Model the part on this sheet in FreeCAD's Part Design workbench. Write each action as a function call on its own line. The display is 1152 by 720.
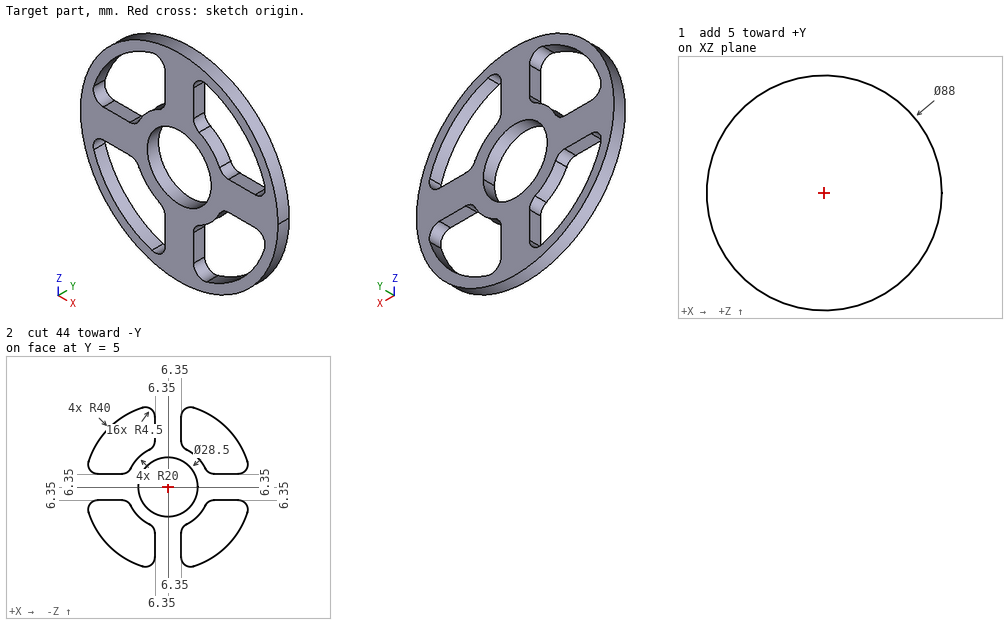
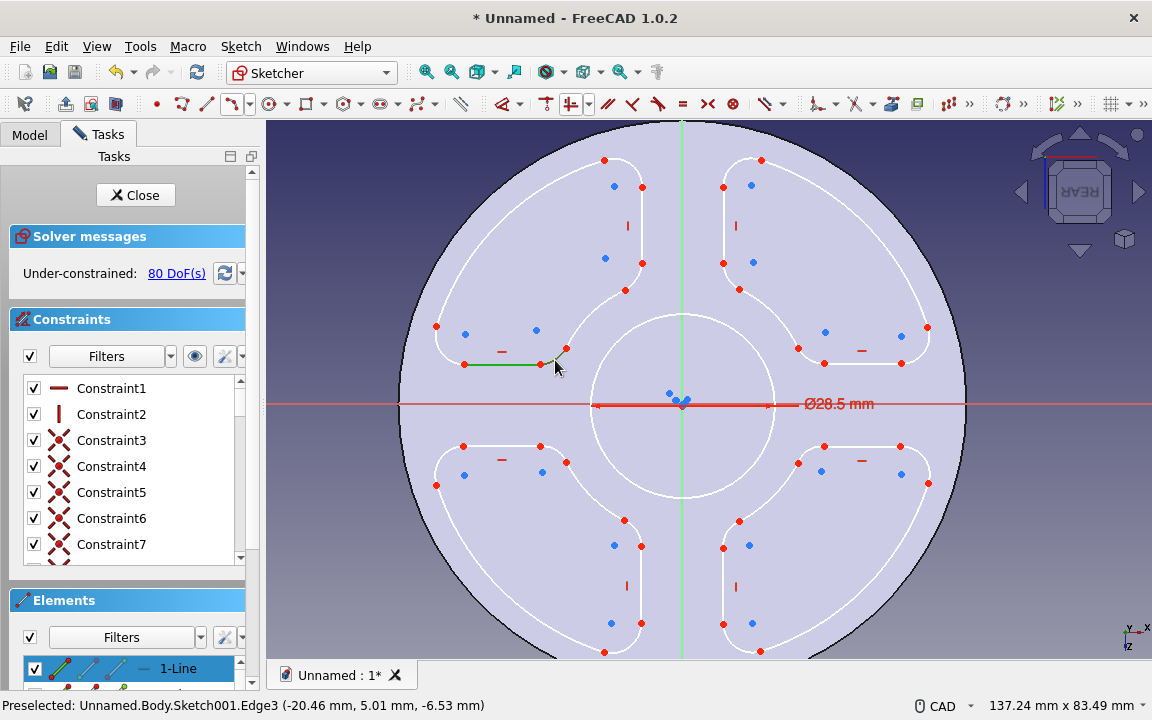
key(t)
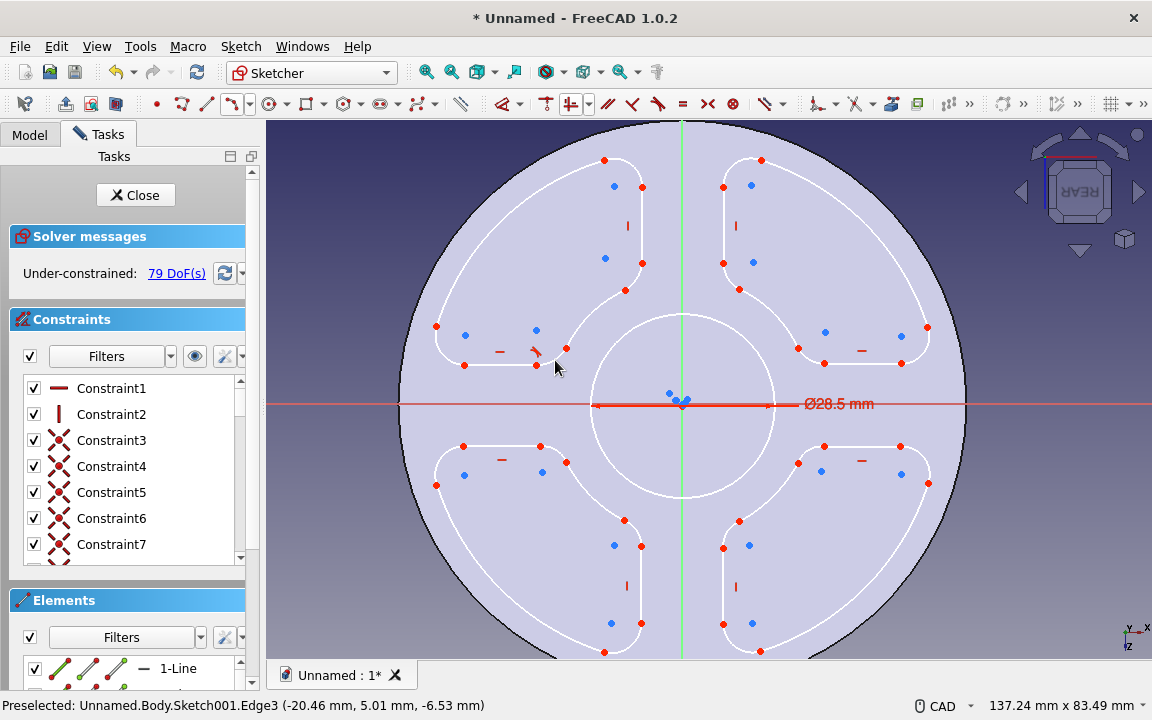
click(486, 365)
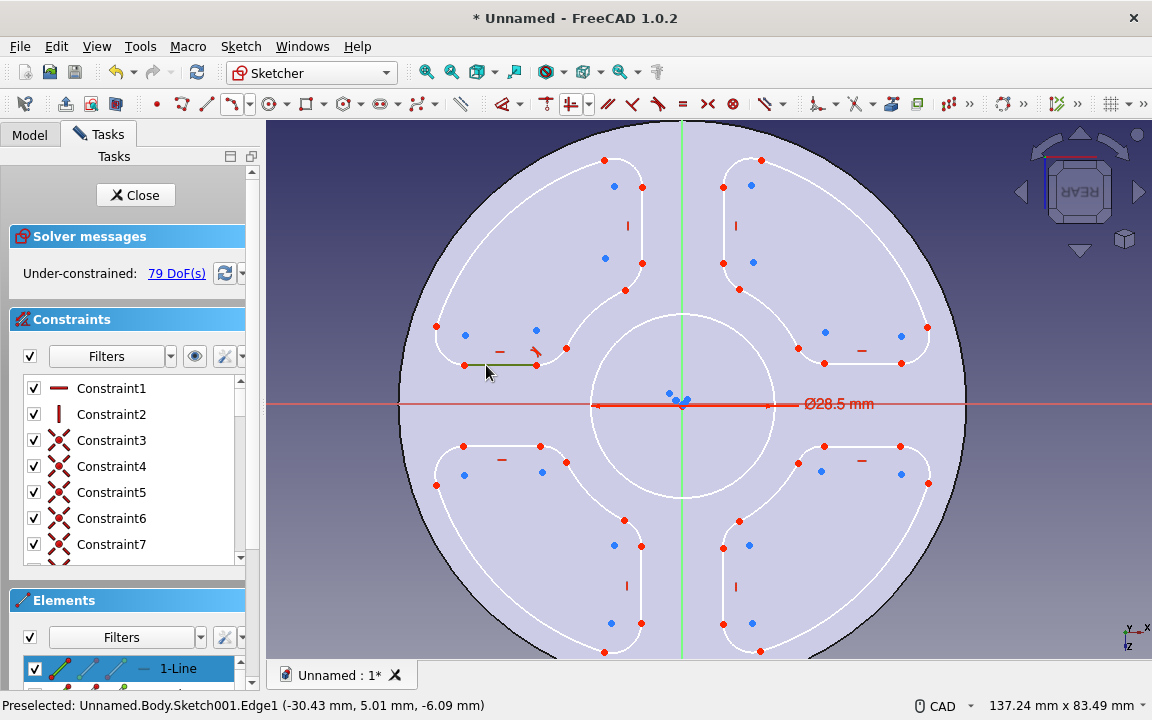
click(437, 343)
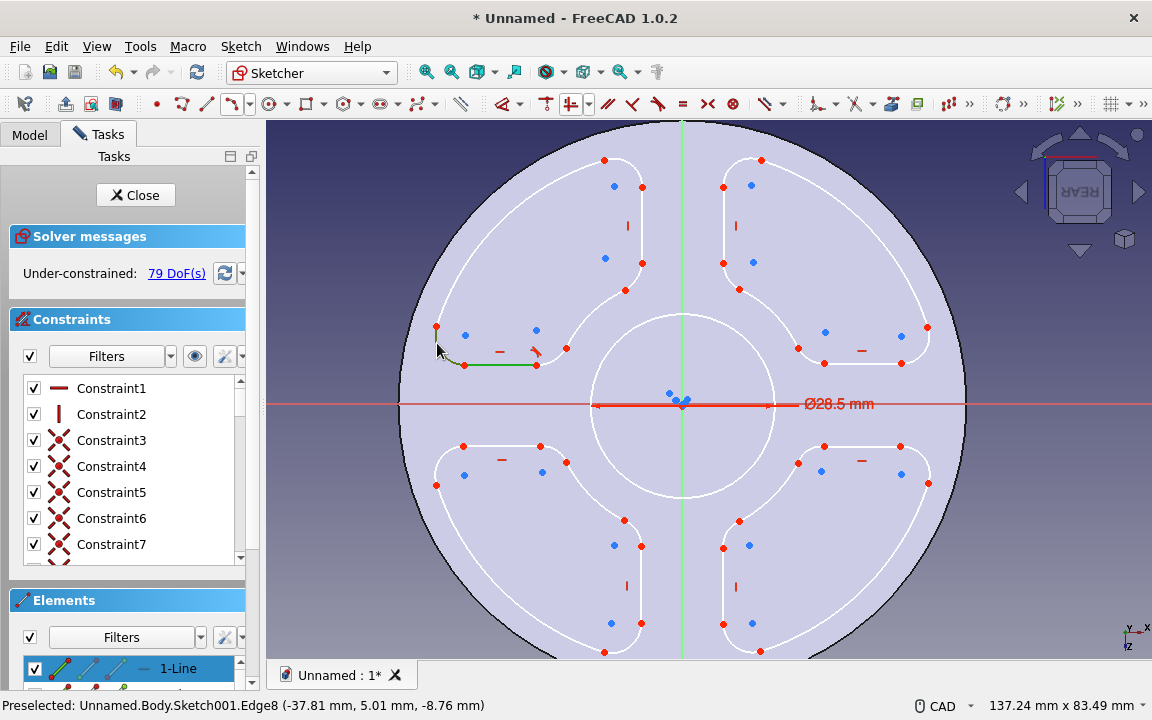
key(t)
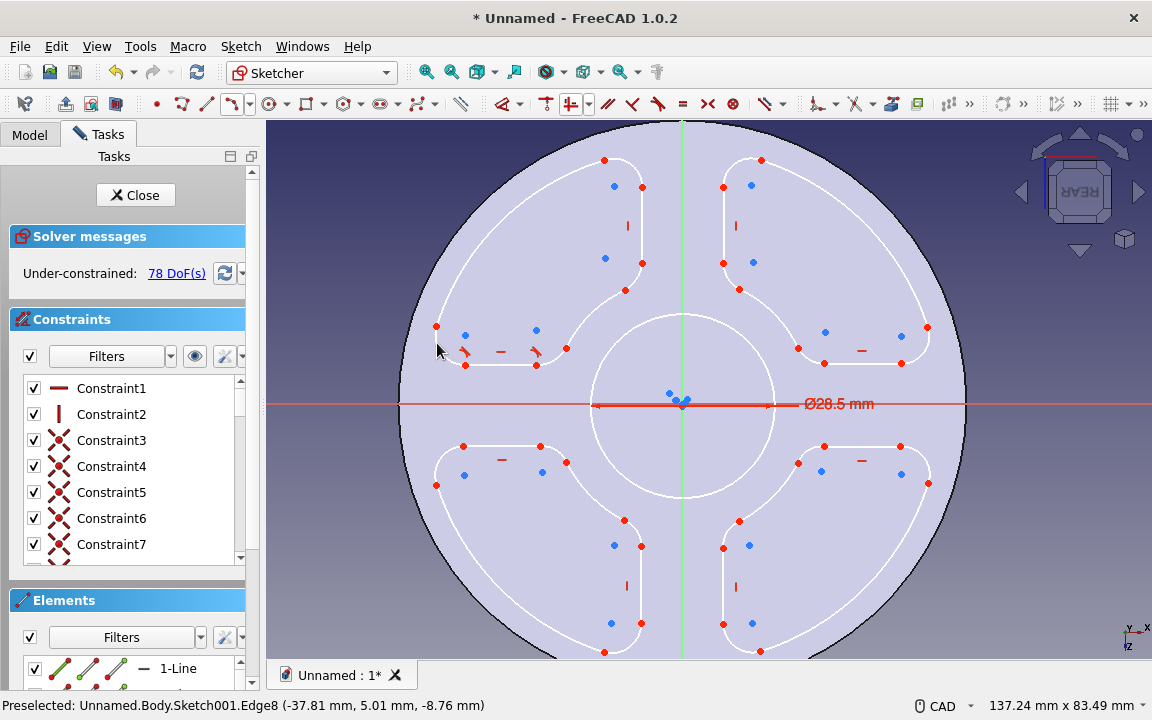
click(642, 241)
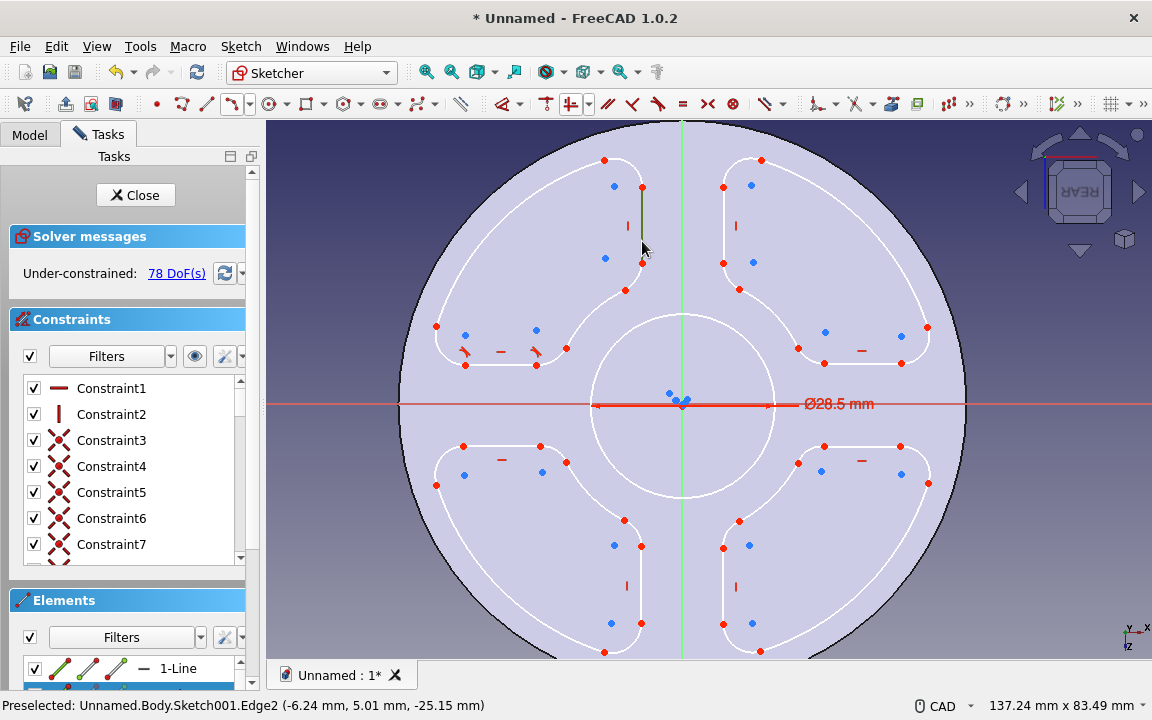
scroll(633, 284, up, 2)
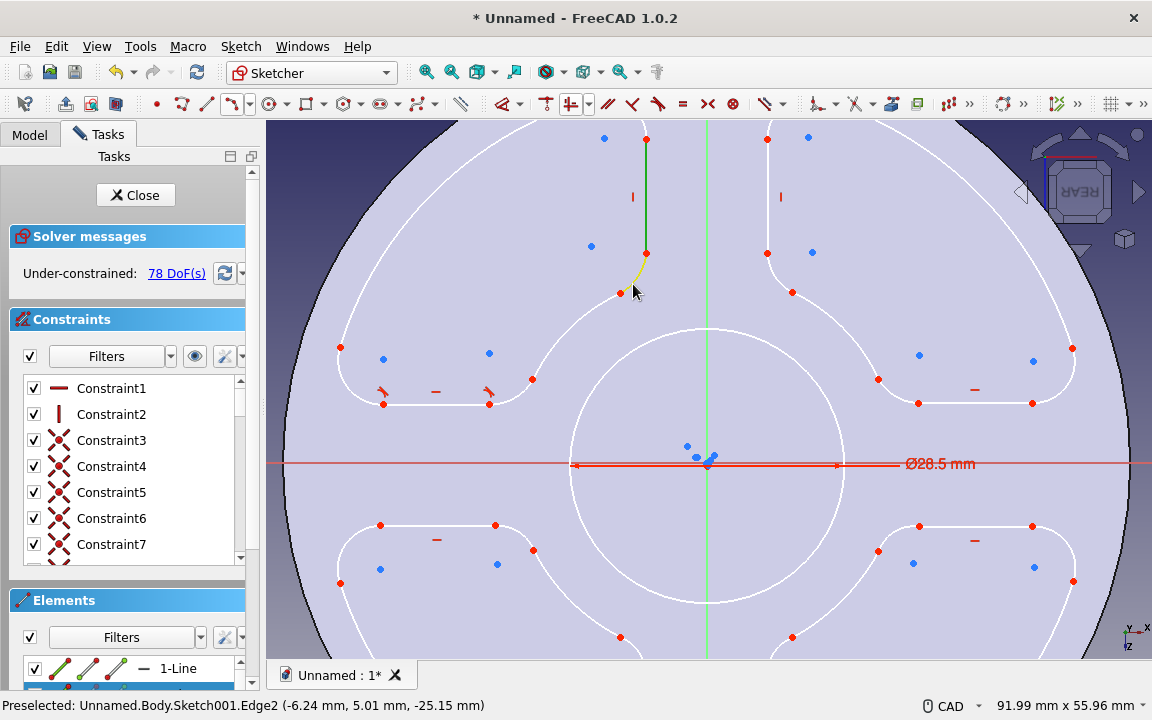
click(632, 284)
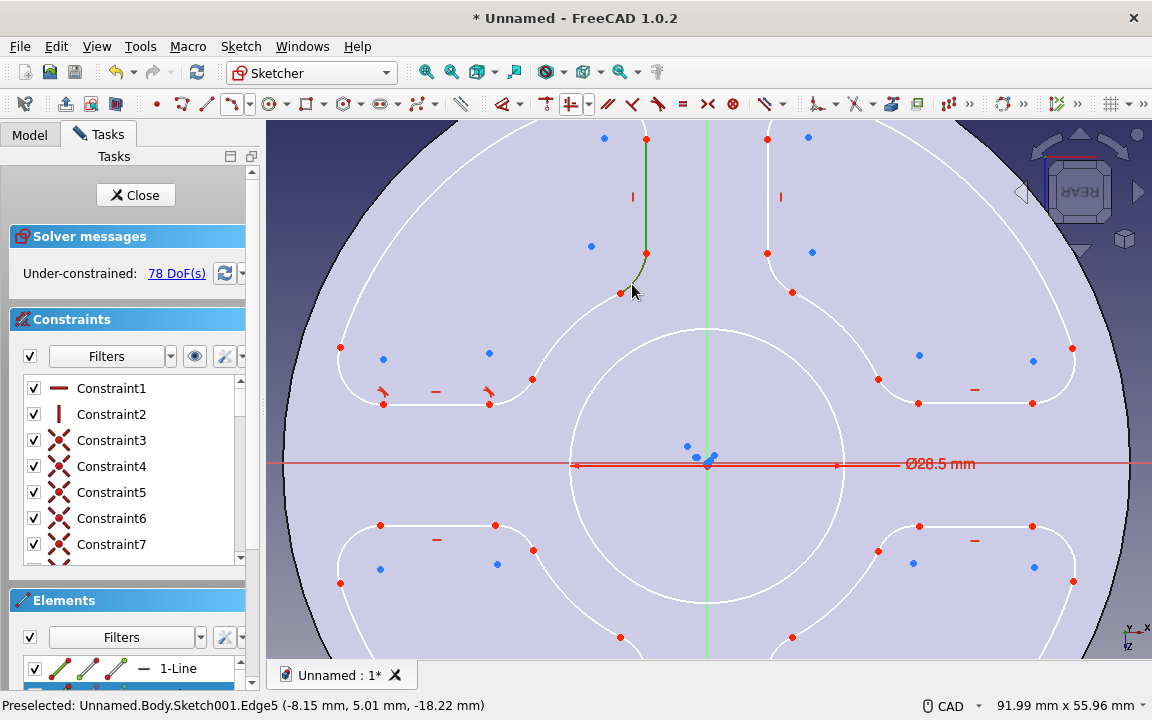
key(t)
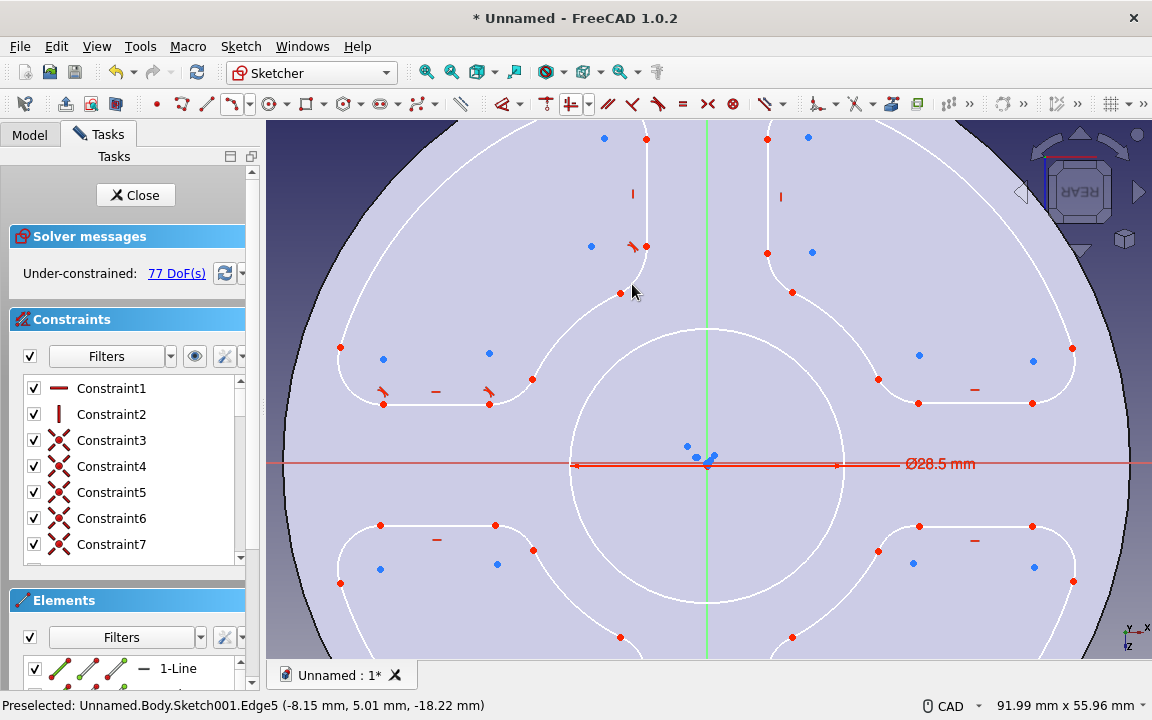
click(647, 214)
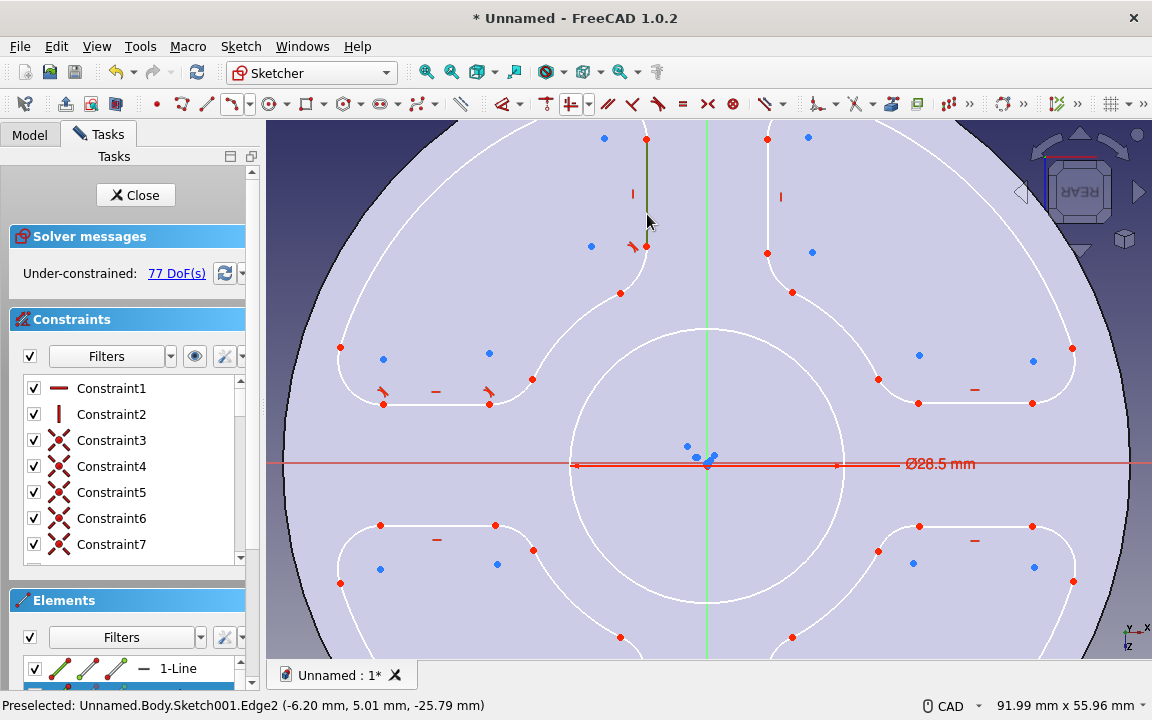
scroll(587, 329, down, 4)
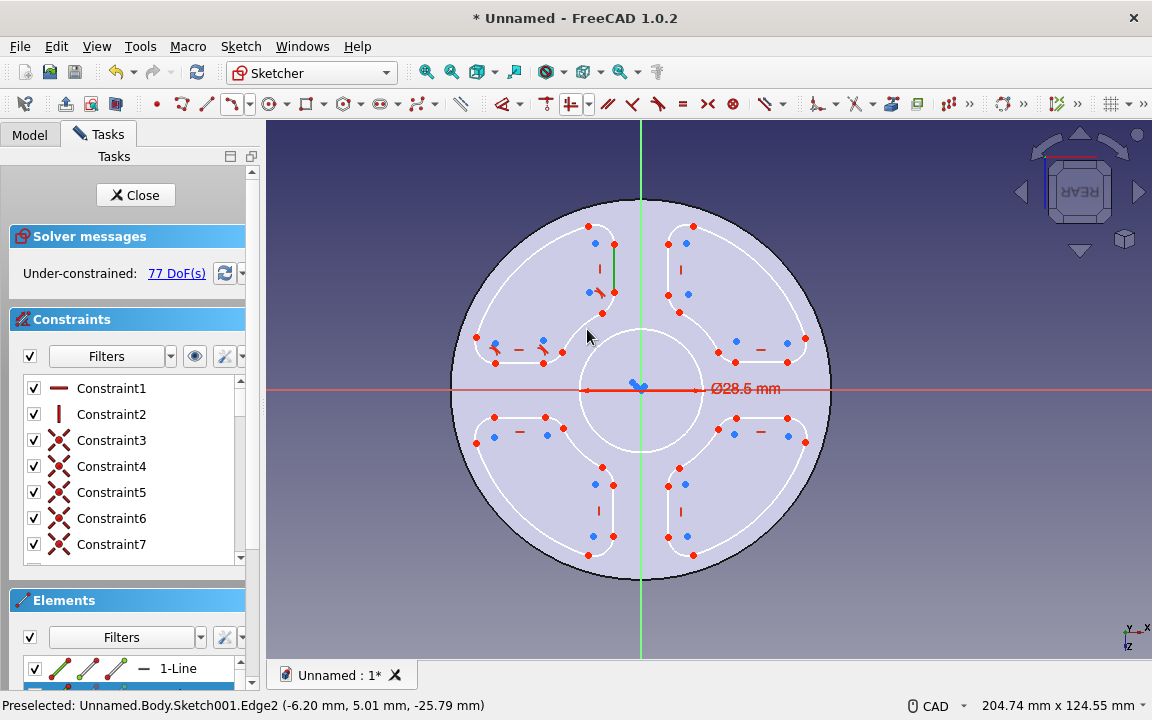
scroll(611, 234, up, 2)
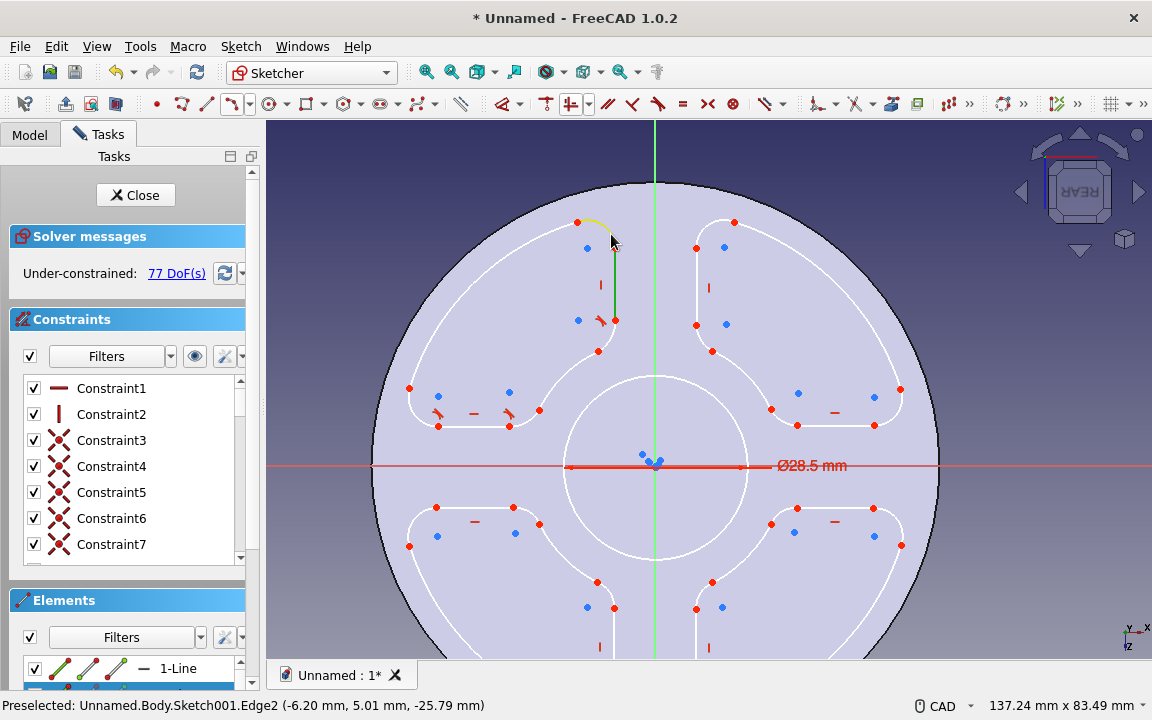
click(611, 233)